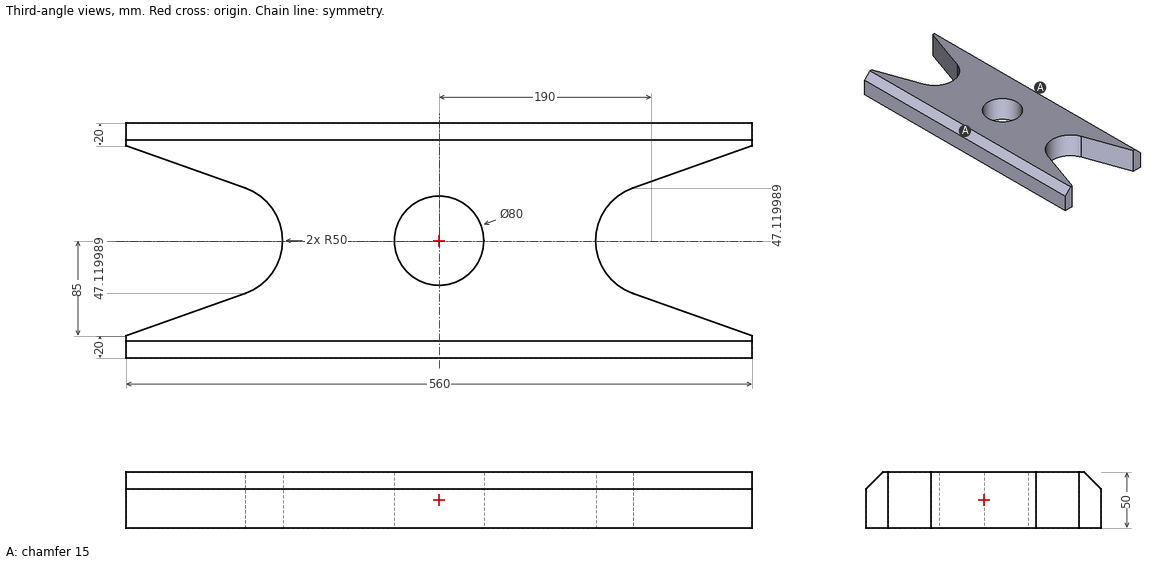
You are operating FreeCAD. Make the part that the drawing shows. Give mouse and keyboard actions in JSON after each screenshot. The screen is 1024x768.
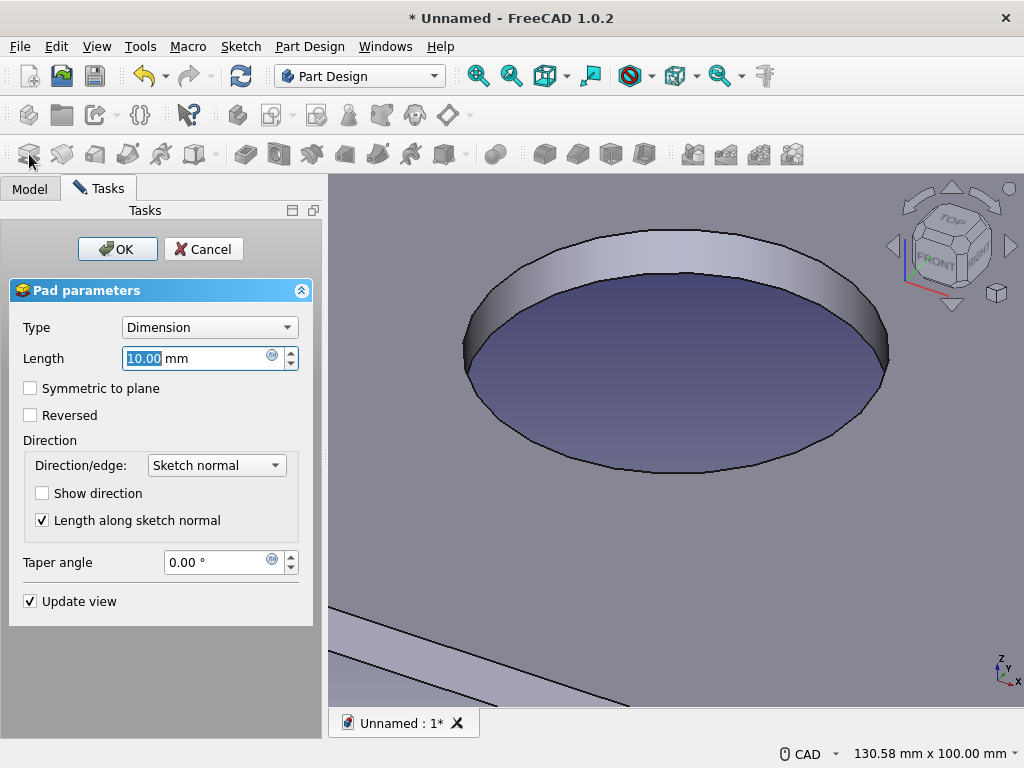
{"action": "type", "text": "50"}
{"action": "key", "text": "Tab"}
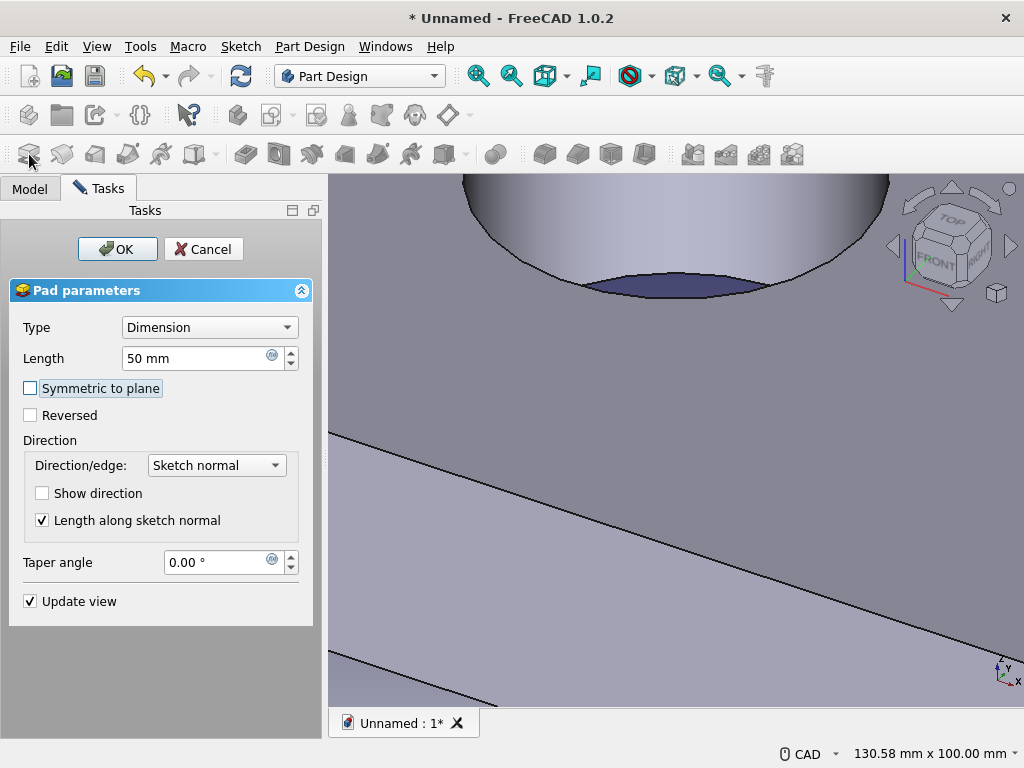
{"action": "left_click", "coordinate": [31, 388]}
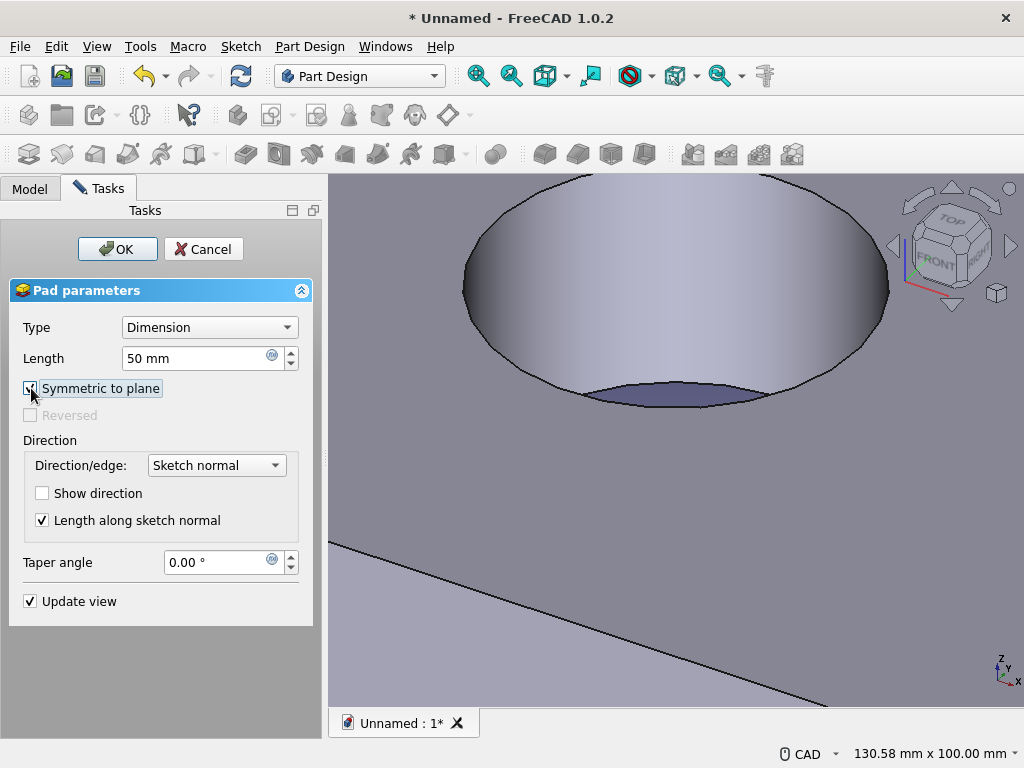
{"action": "left_click", "coordinate": [118, 249]}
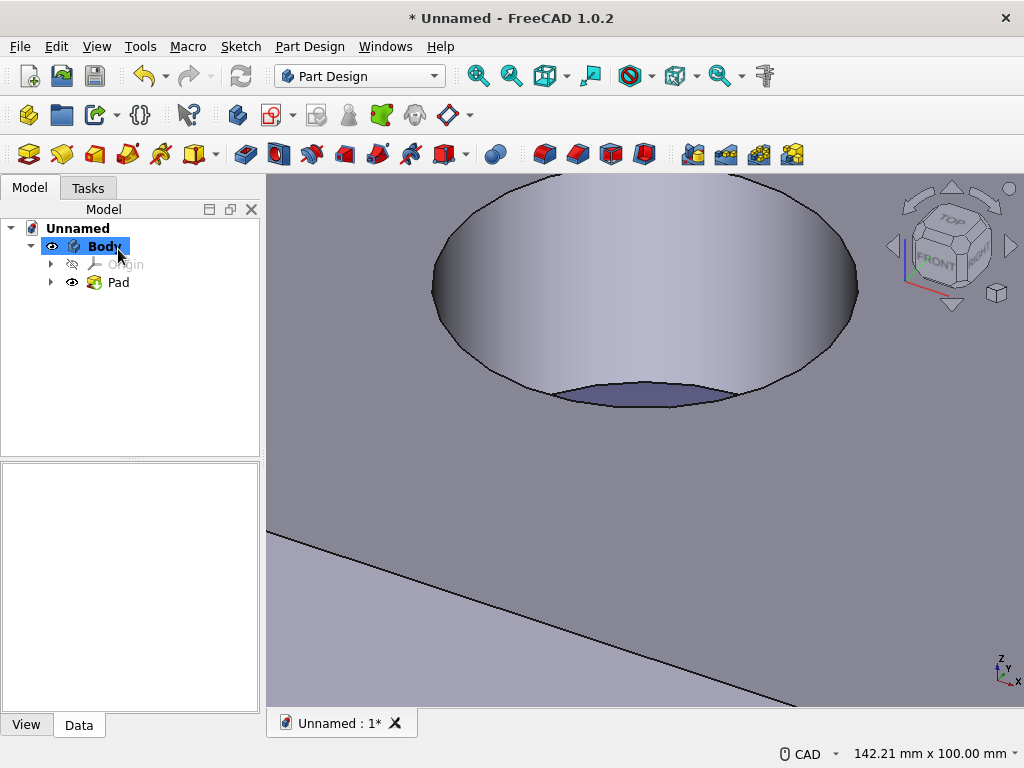
{"action": "key", "text": "v f"}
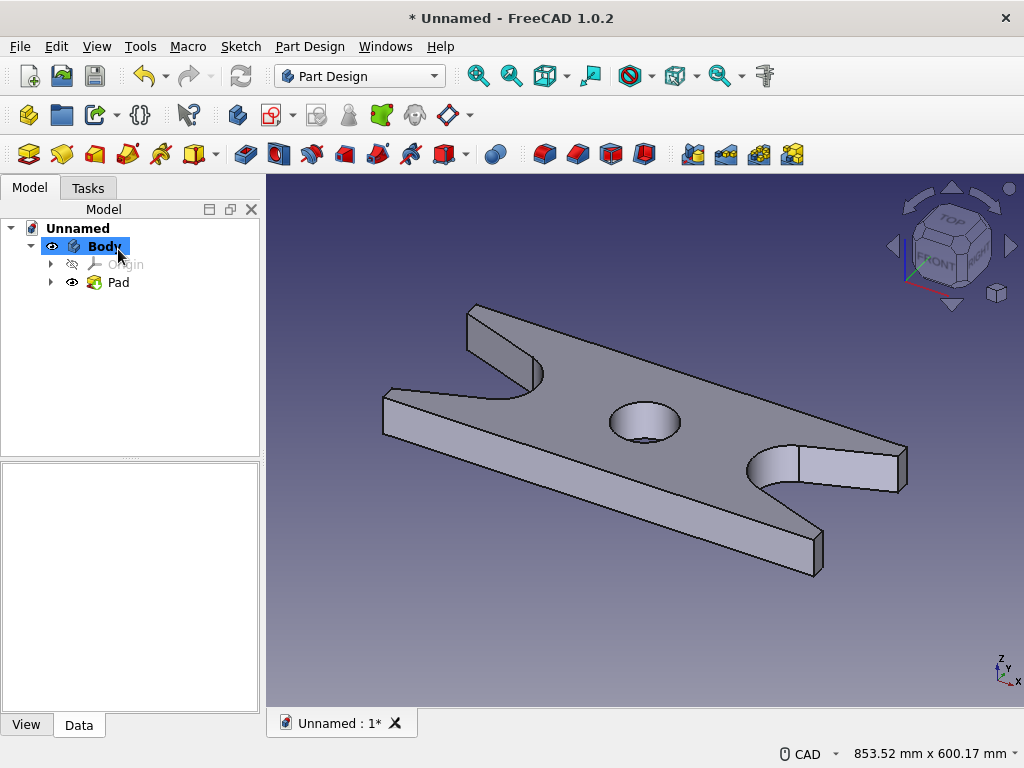
{"action": "left_click", "coordinate": [598, 468]}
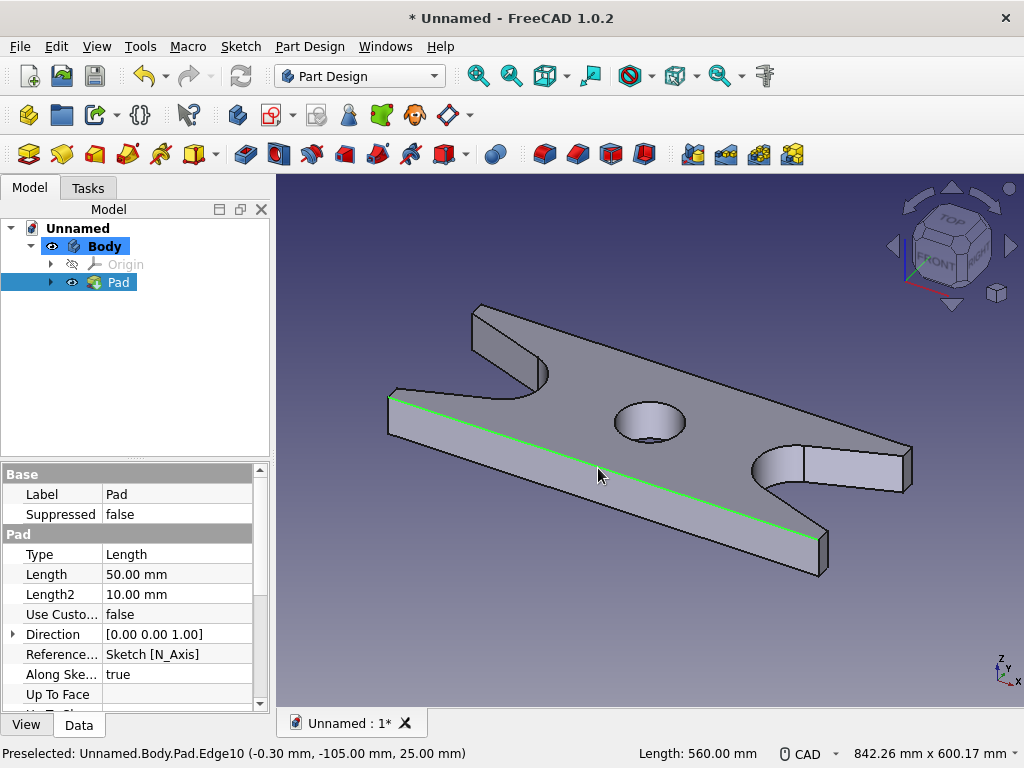
{"action": "key", "text": "0"}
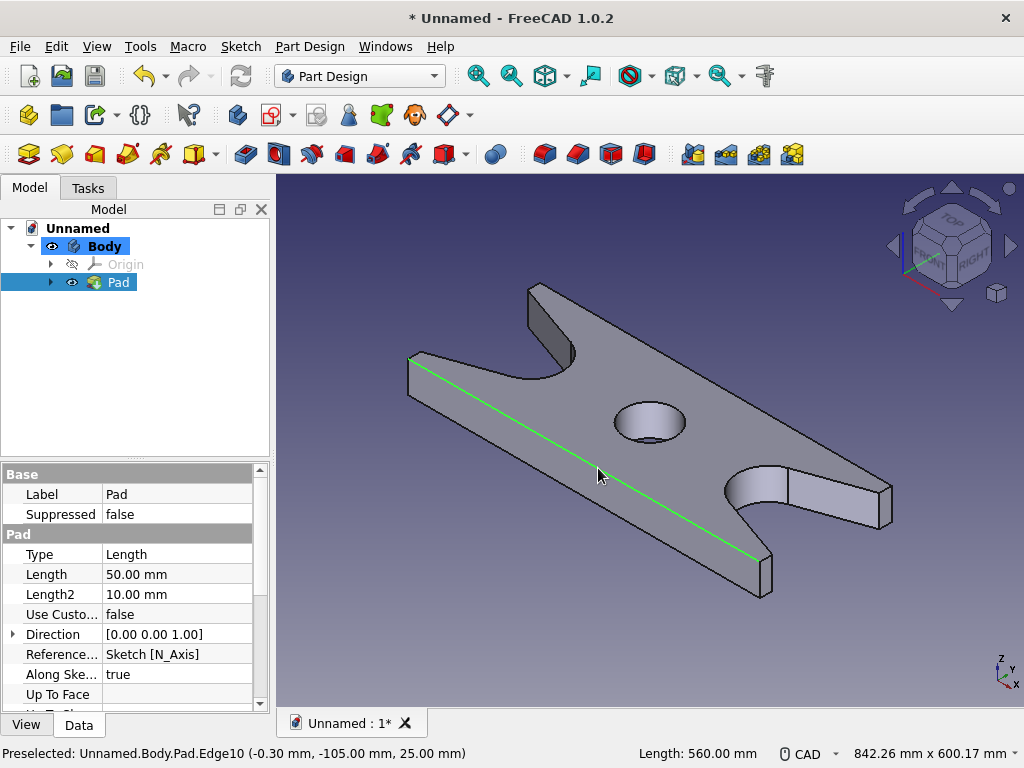
{"action": "key", "text": "2"}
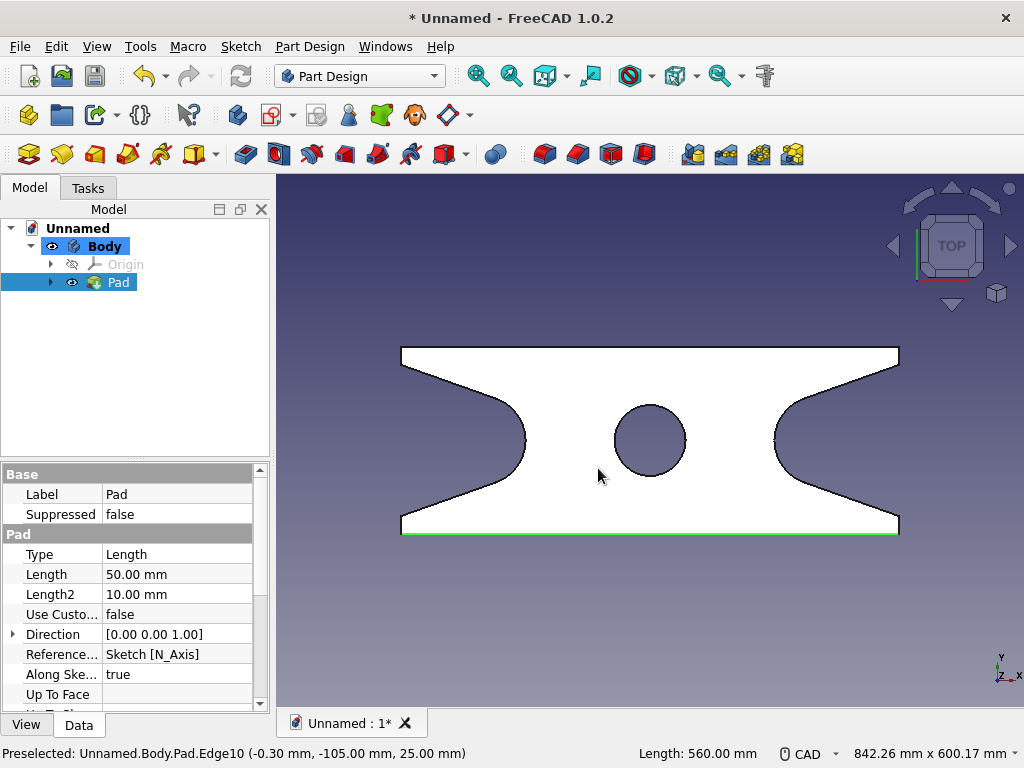
{"action": "left_click", "coordinate": [650, 346], "text": "ctrl"}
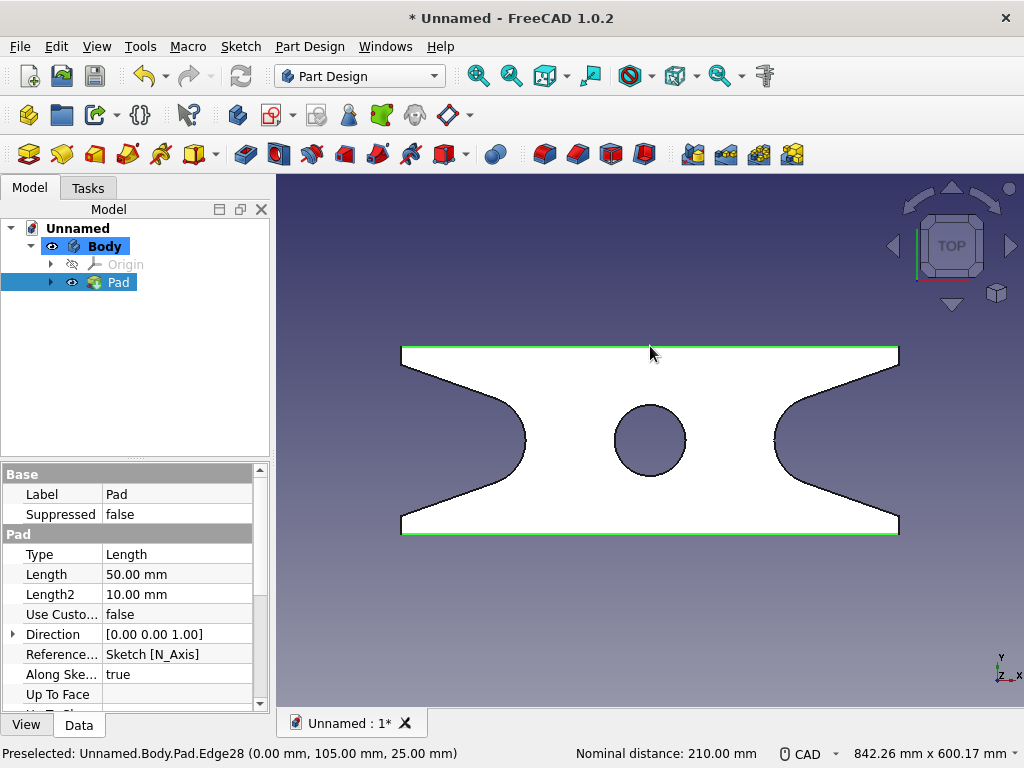
{"action": "left_click", "coordinate": [578, 154]}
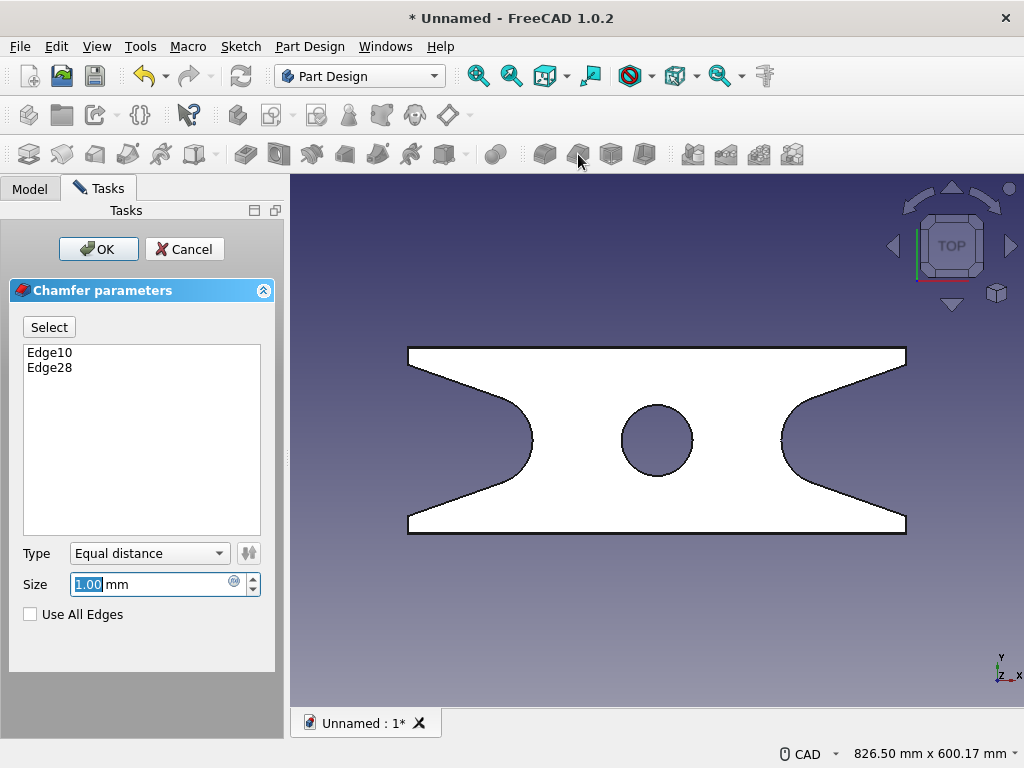
{"action": "type", "text": "15"}
{"action": "key", "text": "Tab"}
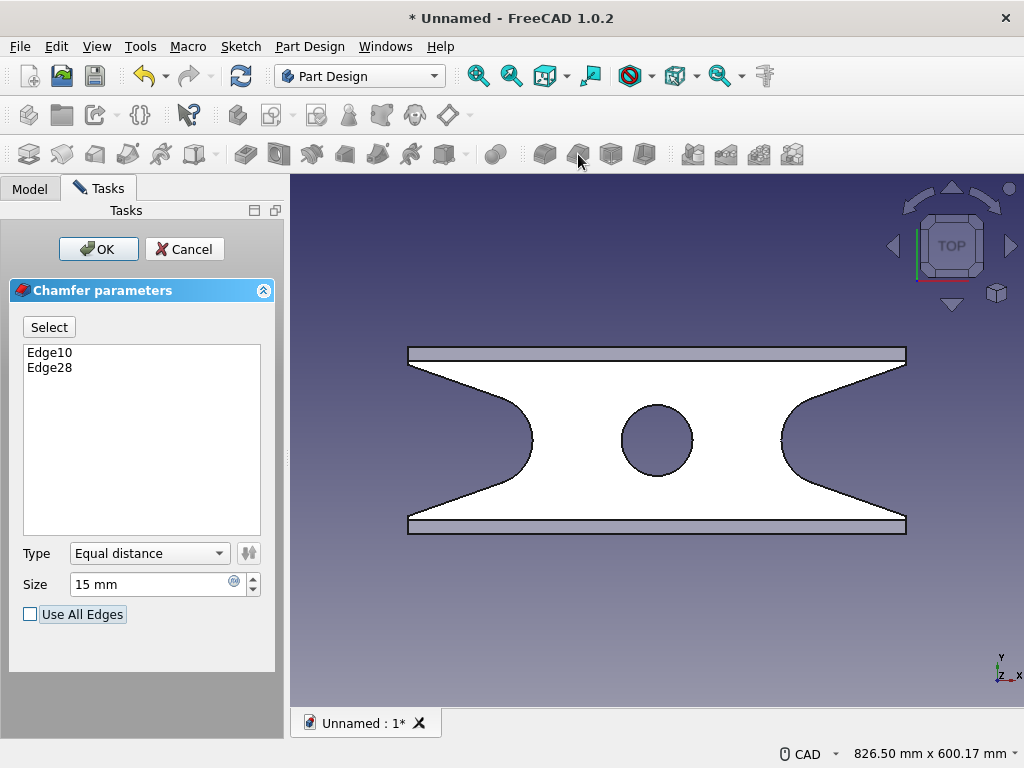
{"action": "left_click", "coordinate": [99, 249]}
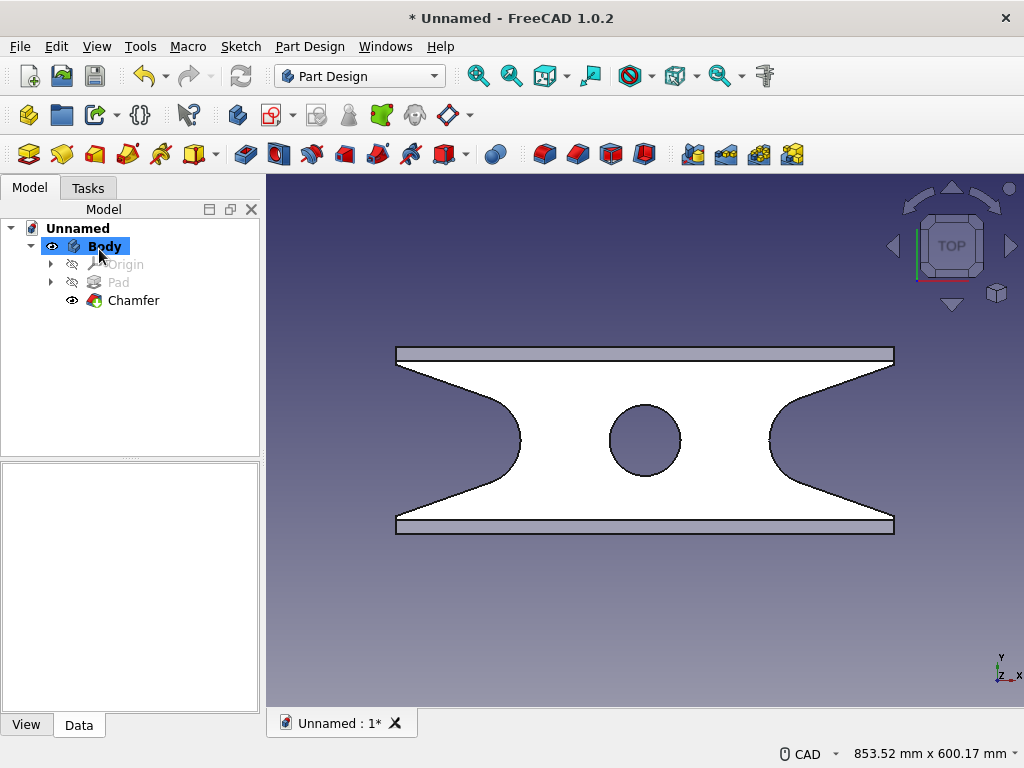
{"action": "key", "text": "0"}